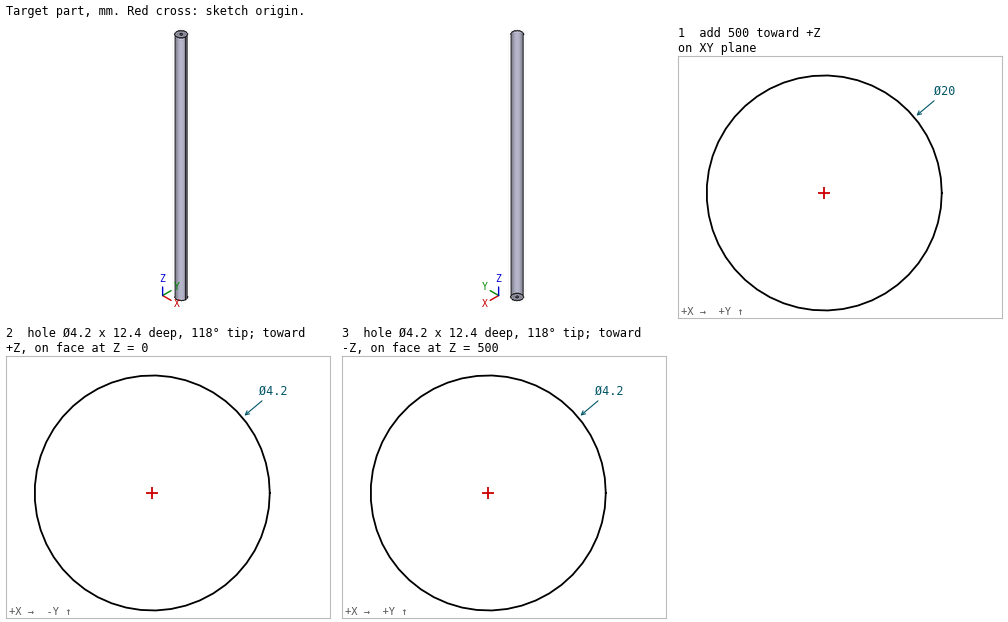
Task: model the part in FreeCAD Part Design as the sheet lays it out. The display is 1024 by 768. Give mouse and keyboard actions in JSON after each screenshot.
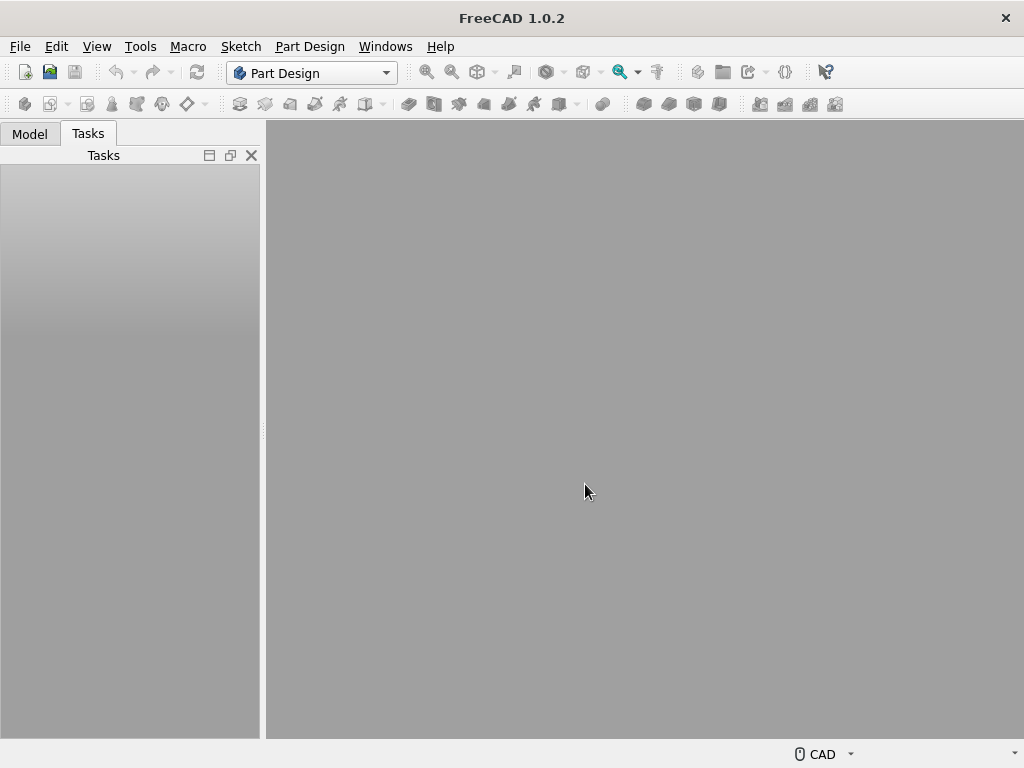
{"action": "left_click", "coordinate": [25, 72]}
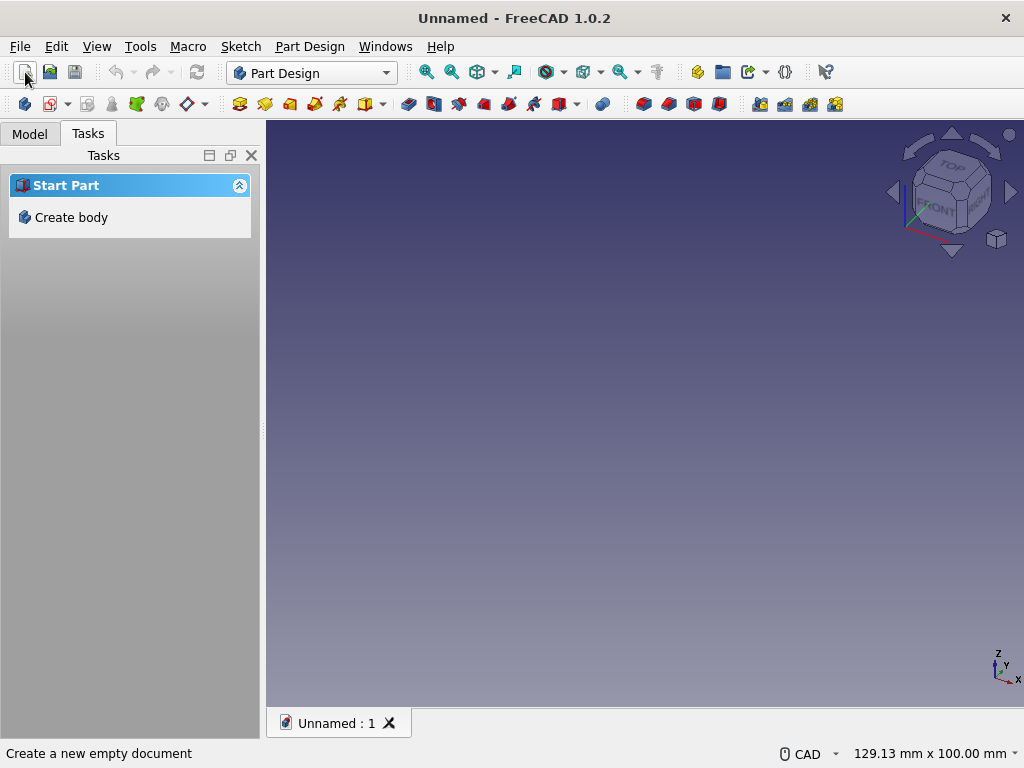
{"action": "left_click", "coordinate": [50, 104]}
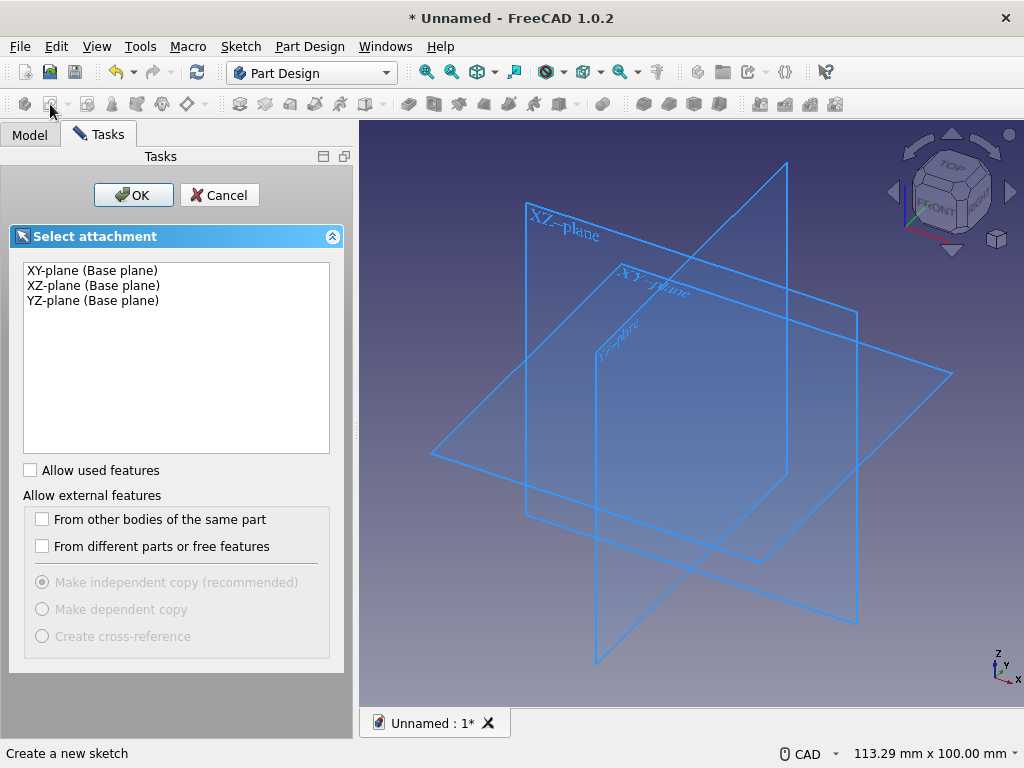
{"action": "left_click", "coordinate": [84, 270]}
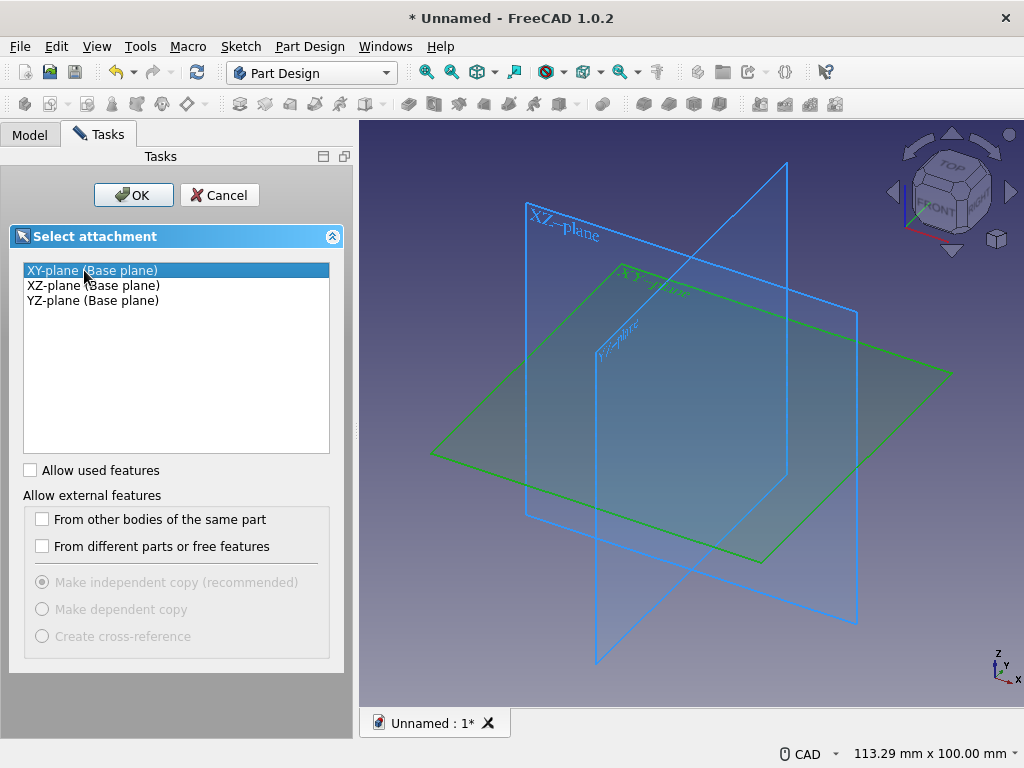
{"action": "left_click", "coordinate": [134, 195]}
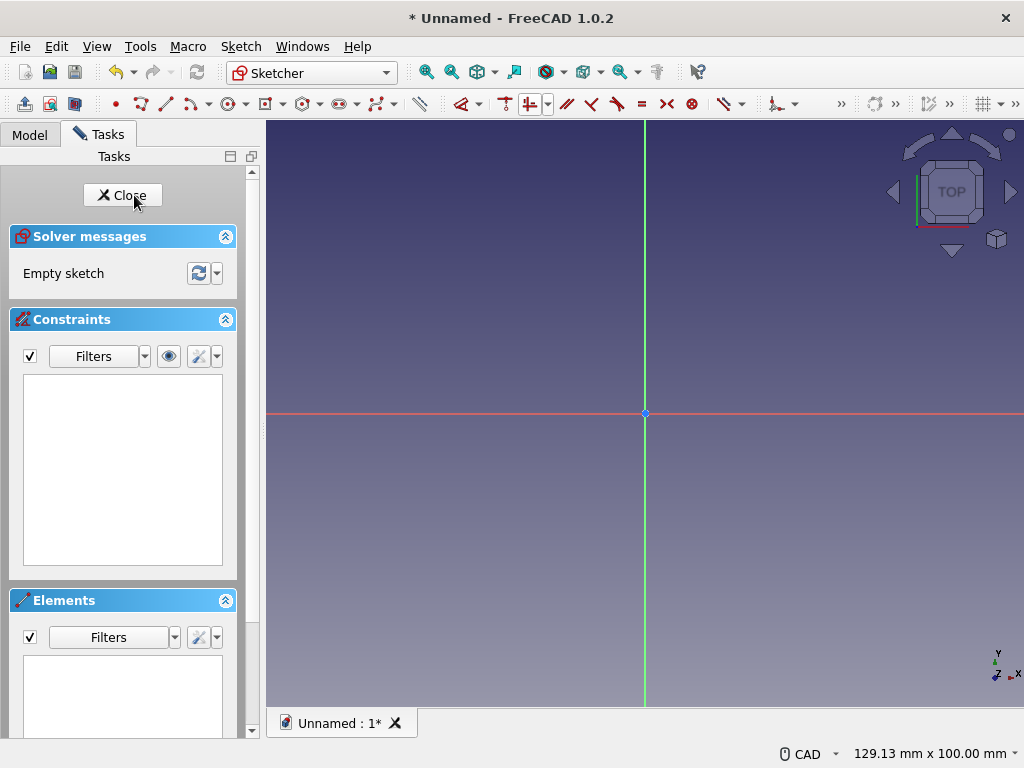
{"action": "scroll", "coordinate": [675, 414], "scroll_direction": "up", "scroll_amount": 6}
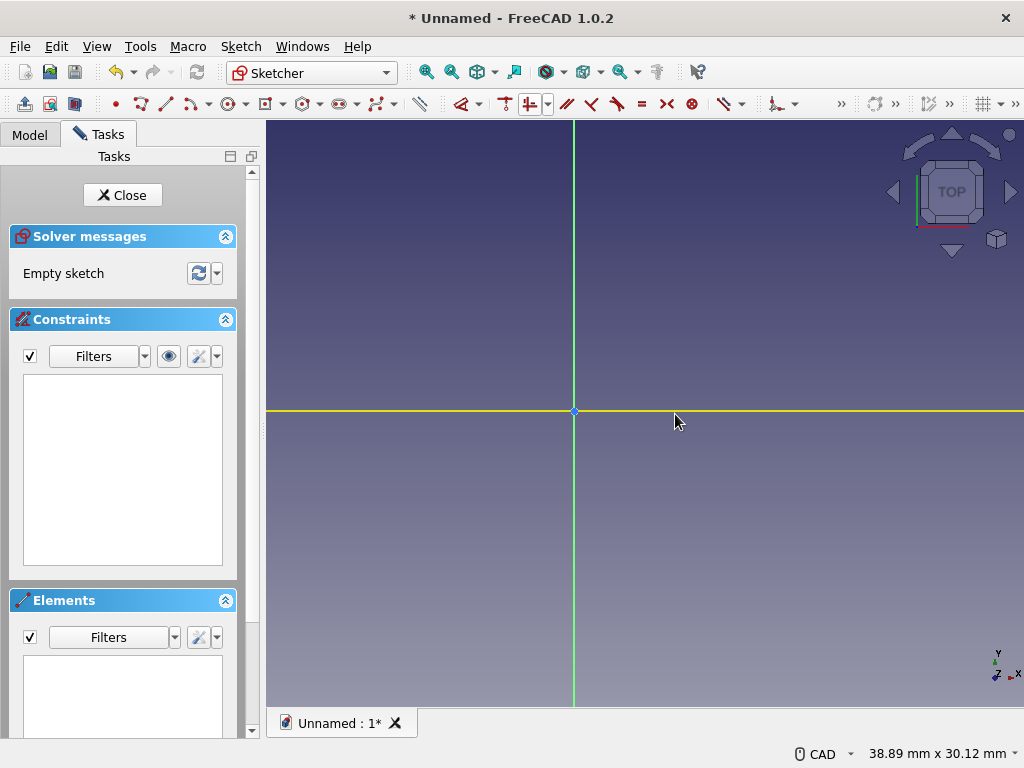
{"action": "key", "text": "g c"}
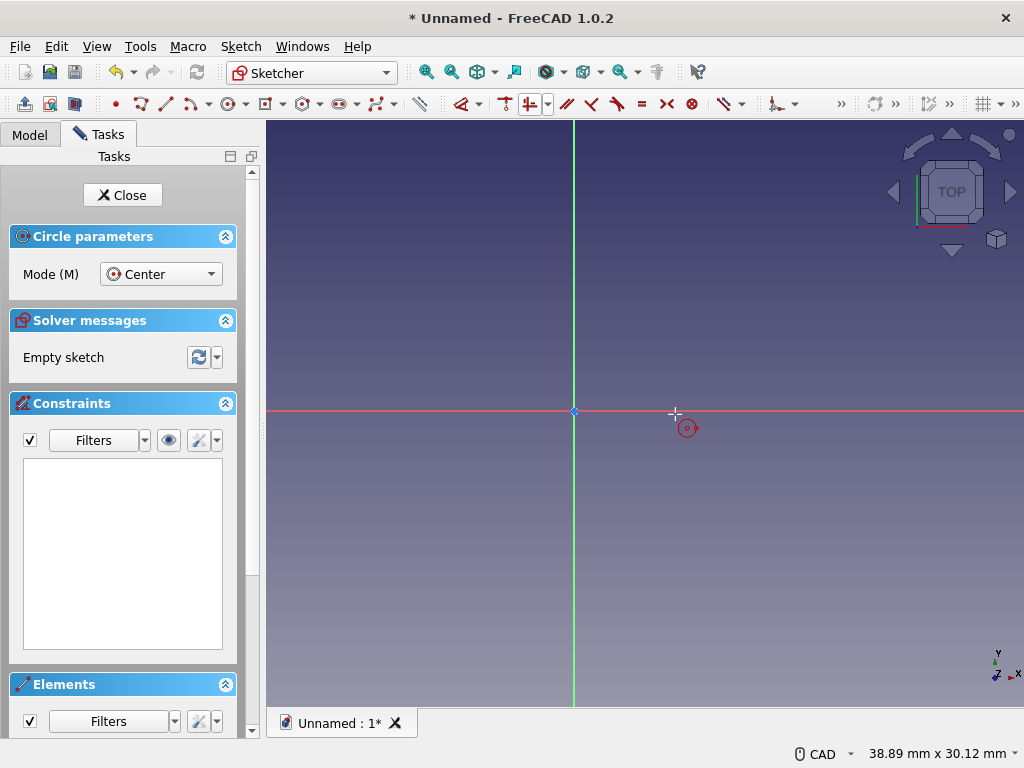
{"action": "left_click", "coordinate": [574, 411]}
{"action": "left_click", "coordinate": [712, 273]}
{"action": "key", "text": "Escape"}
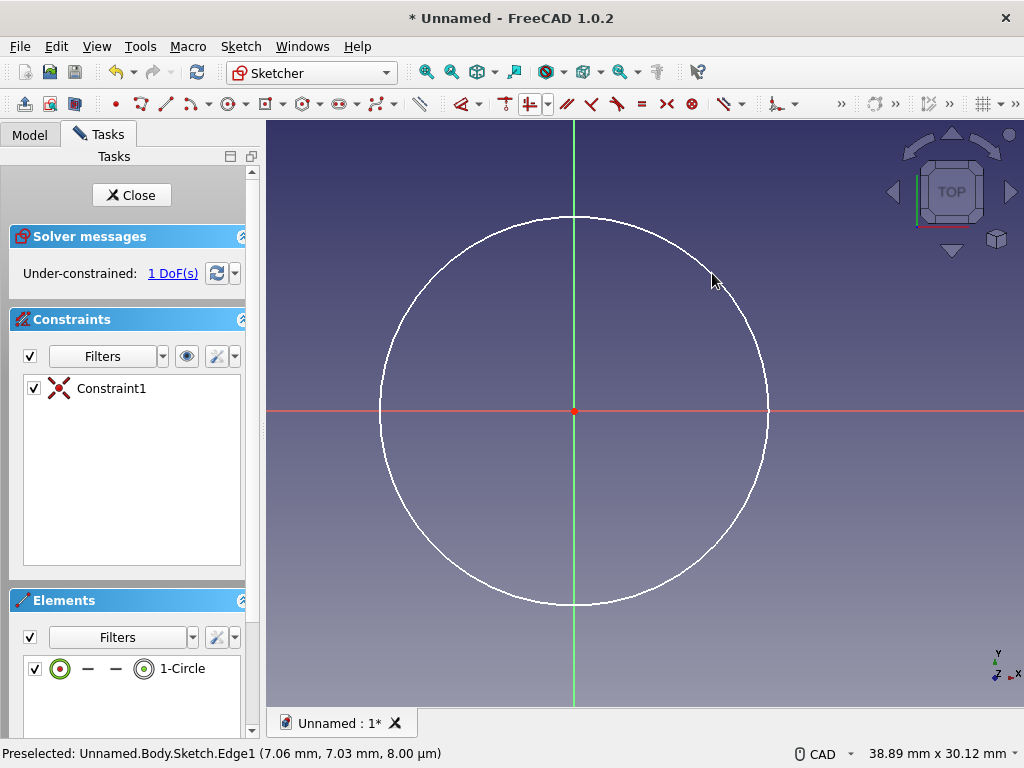
{"action": "left_click", "coordinate": [711, 273]}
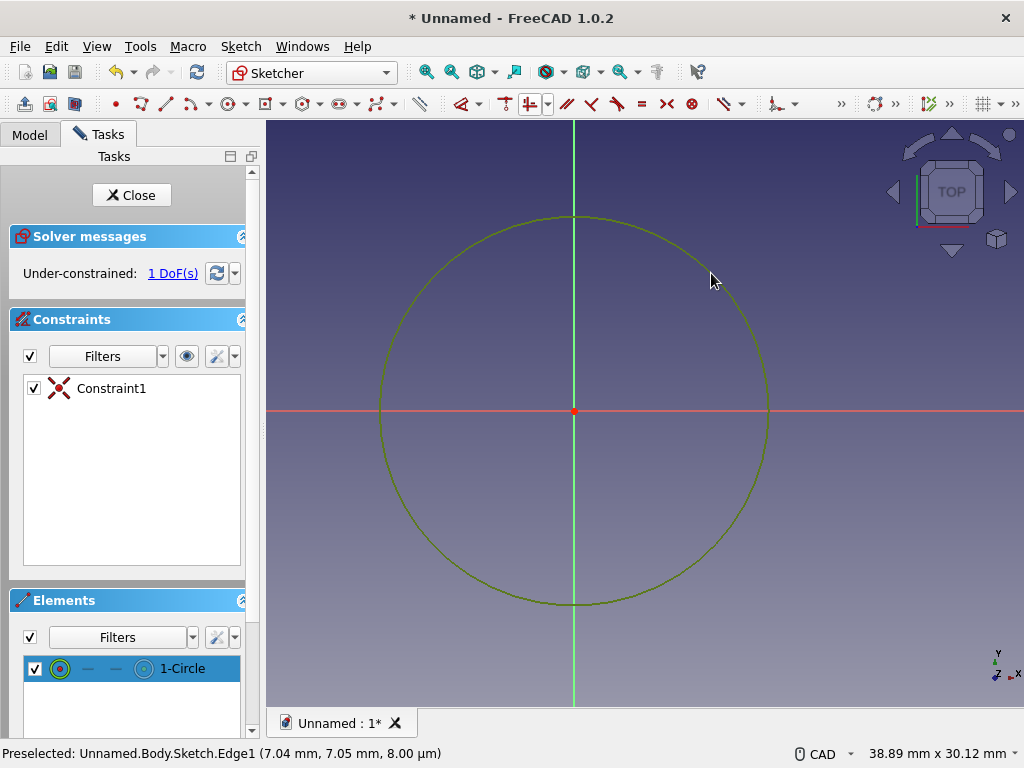
{"action": "key", "text": "k o"}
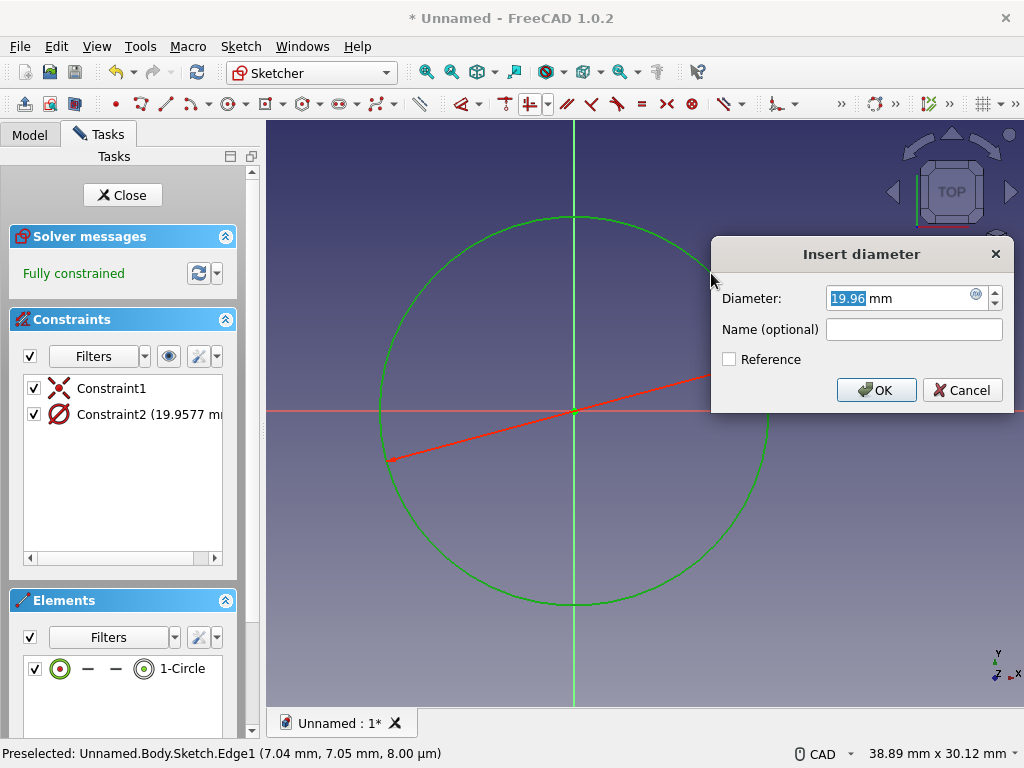
{"action": "type", "text": "20"}
{"action": "key", "text": "Return"}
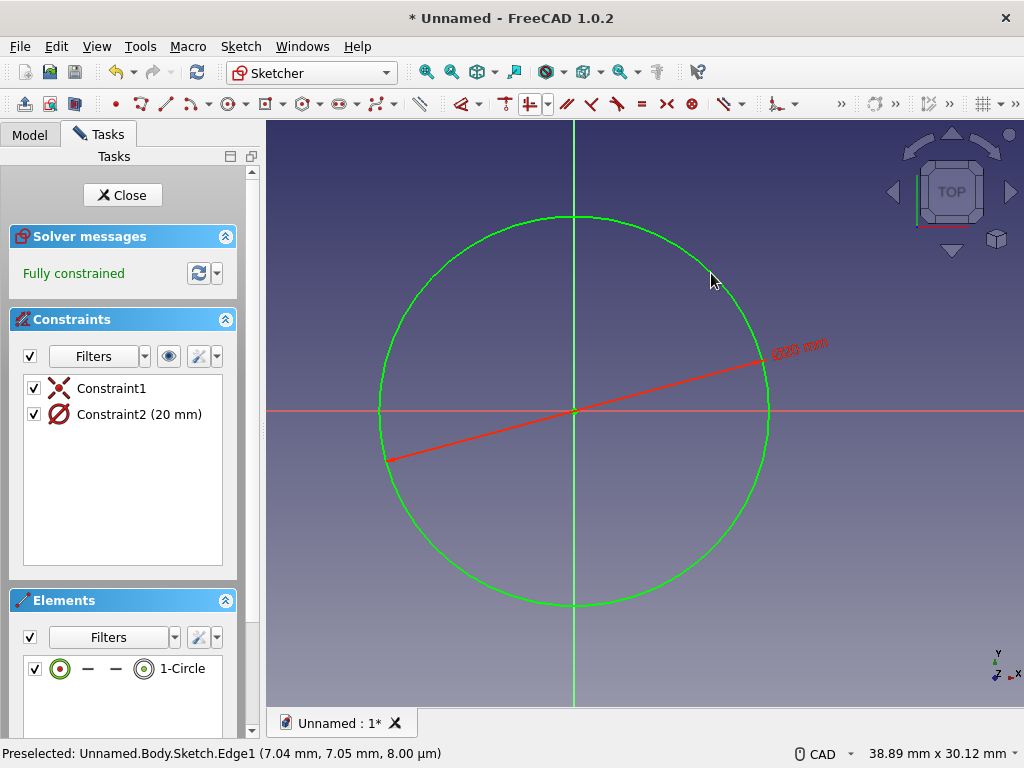
{"action": "left_click", "coordinate": [123, 195]}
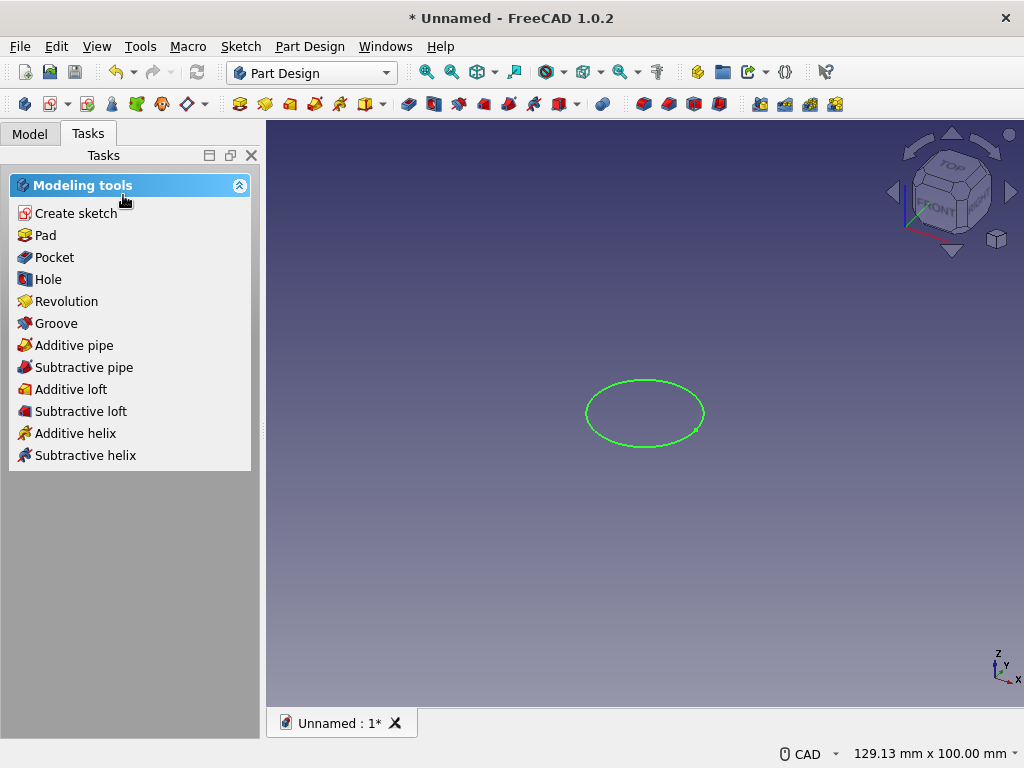
{"action": "left_click", "coordinate": [240, 104]}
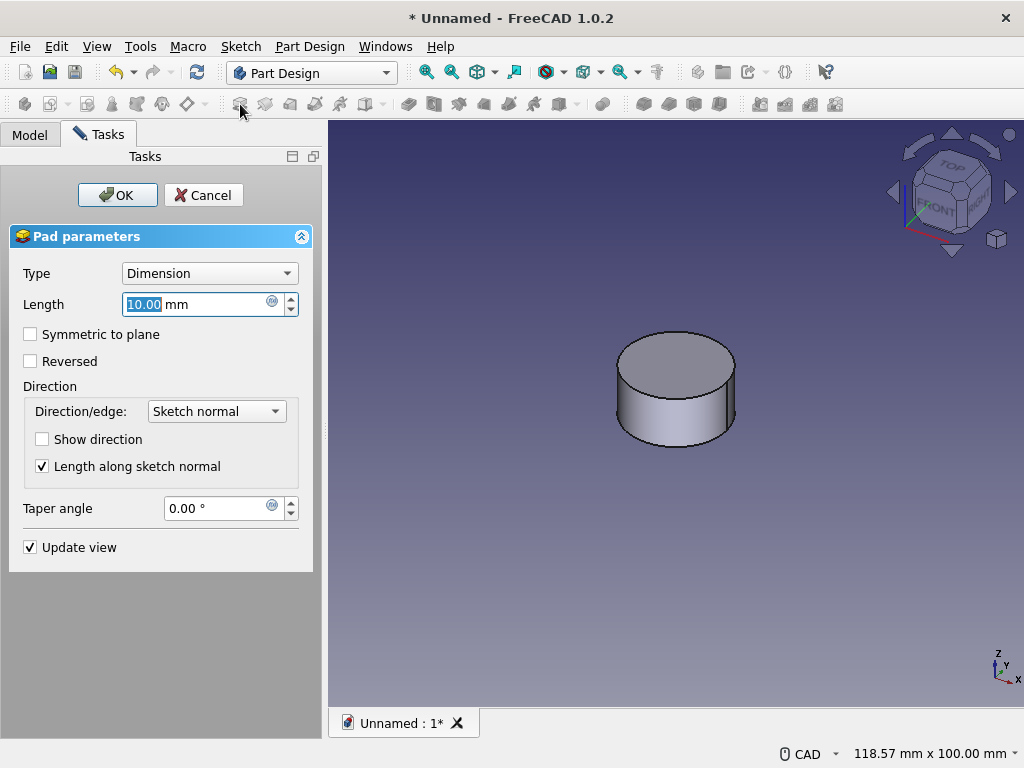
{"action": "type", "text": "500"}
{"action": "key", "text": "Tab"}